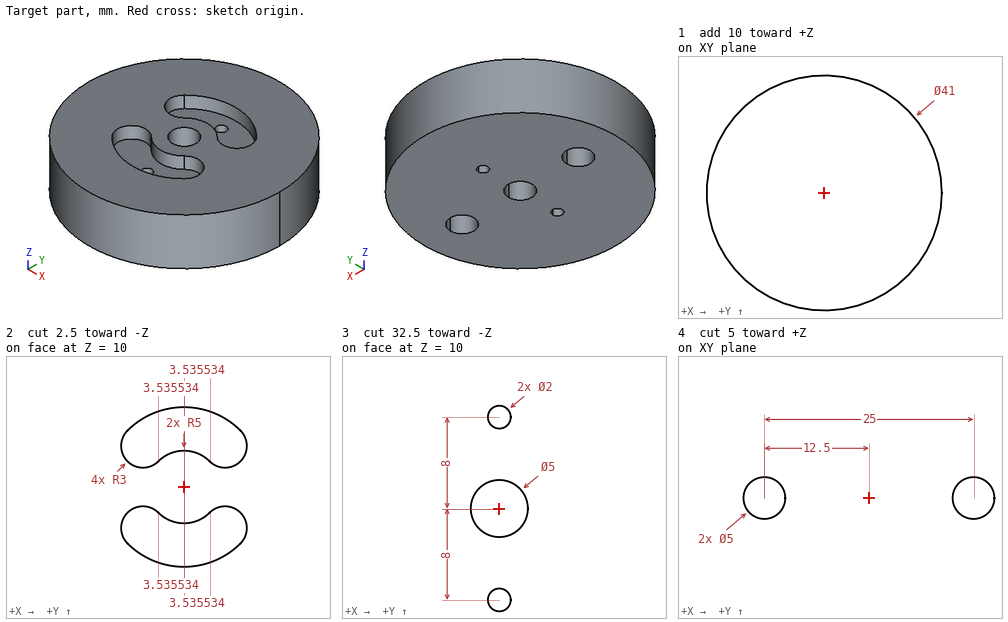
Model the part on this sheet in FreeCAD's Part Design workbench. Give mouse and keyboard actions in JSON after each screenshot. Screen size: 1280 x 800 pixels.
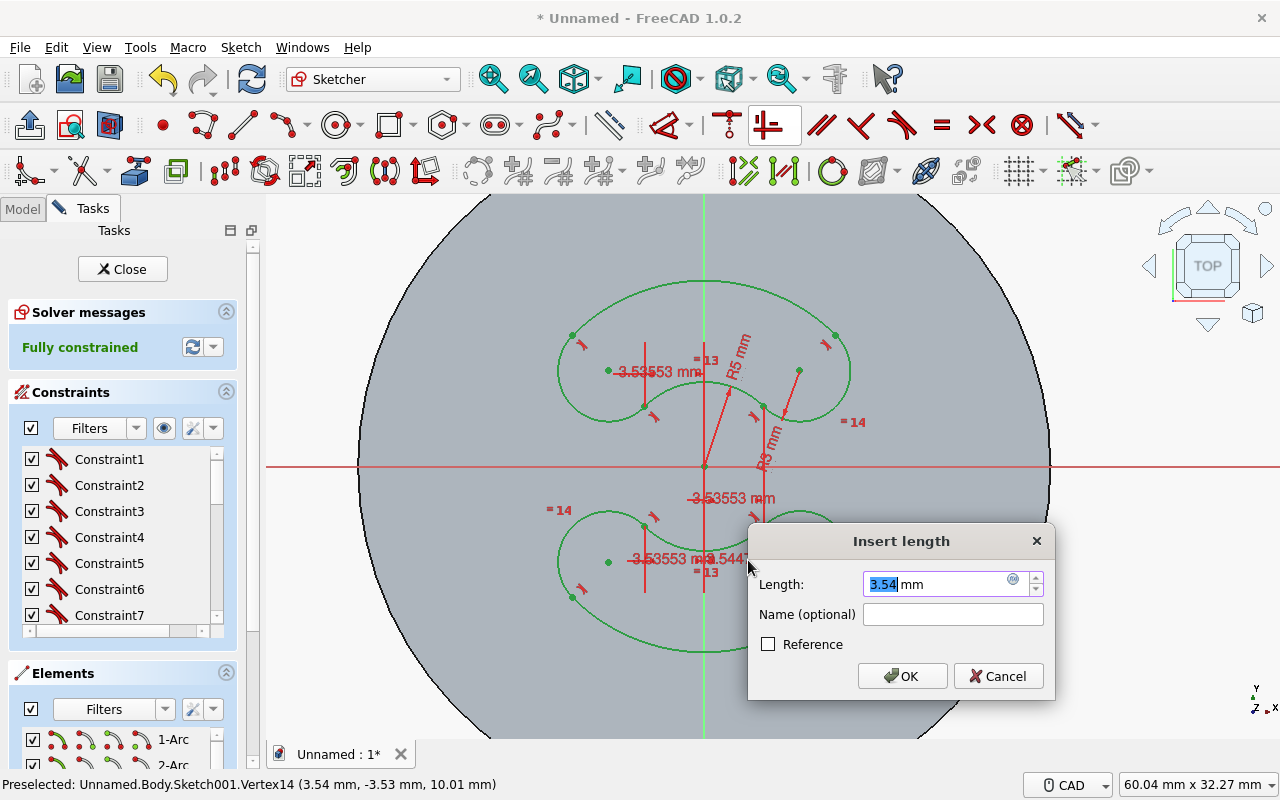
{"action": "type", "text": "3.535534"}
{"action": "key", "text": "Return"}
{"action": "key", "text": "Escape"}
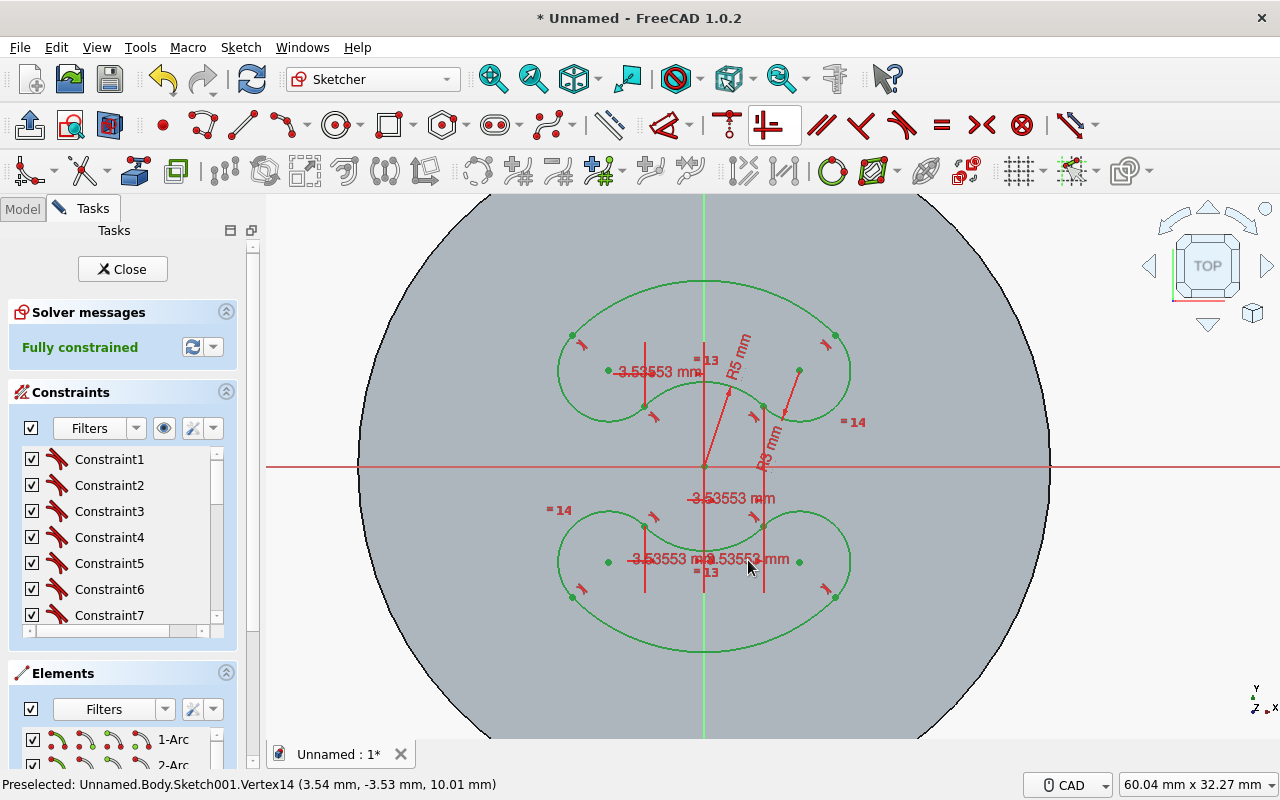
{"action": "left_click", "coordinate": [123, 269]}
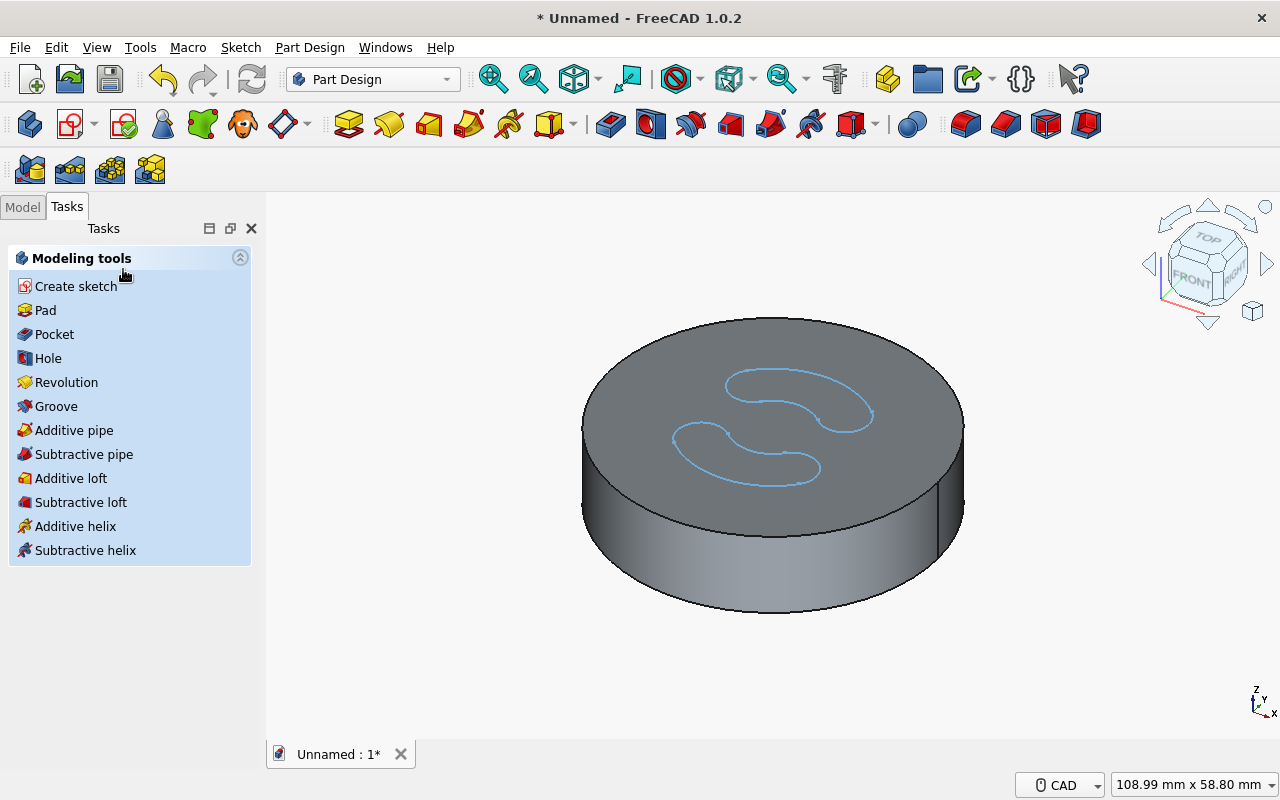
{"action": "left_click", "coordinate": [612, 124]}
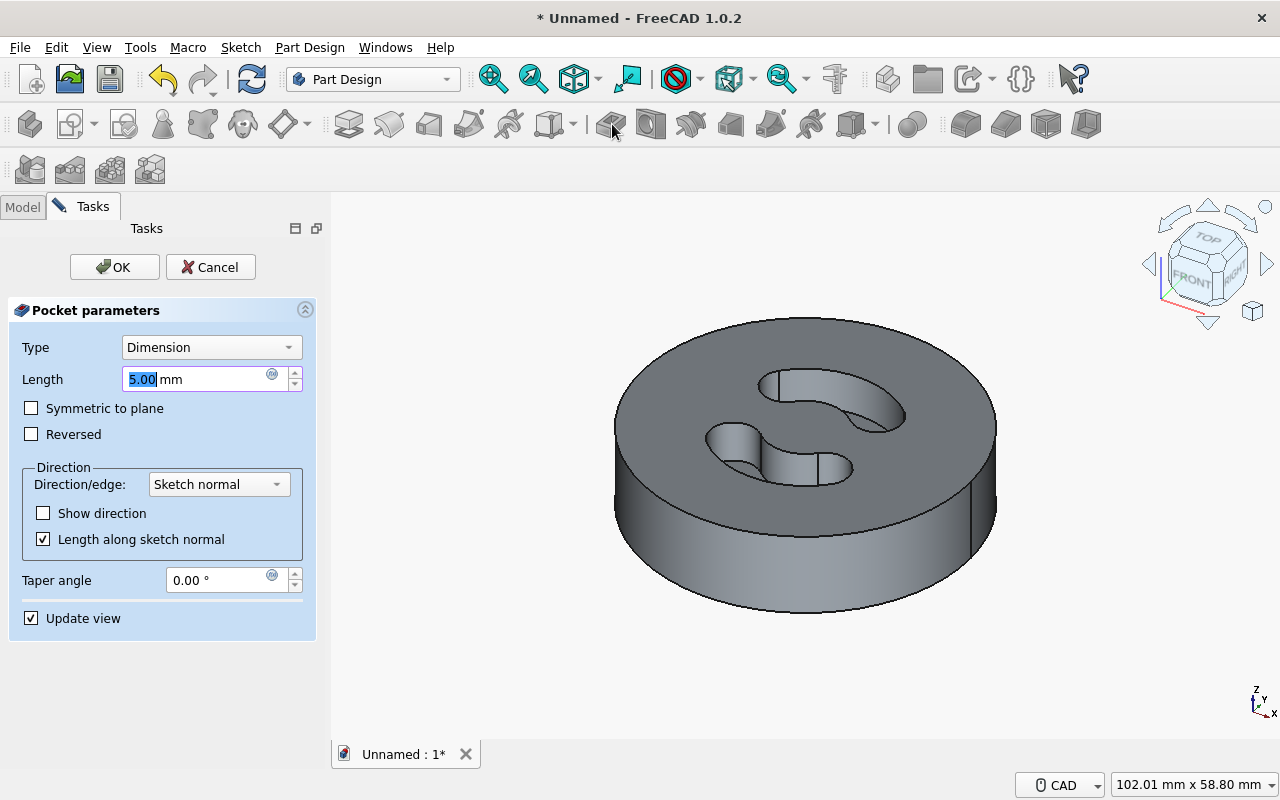
{"action": "type", "text": "2.5"}
{"action": "key", "text": "Tab"}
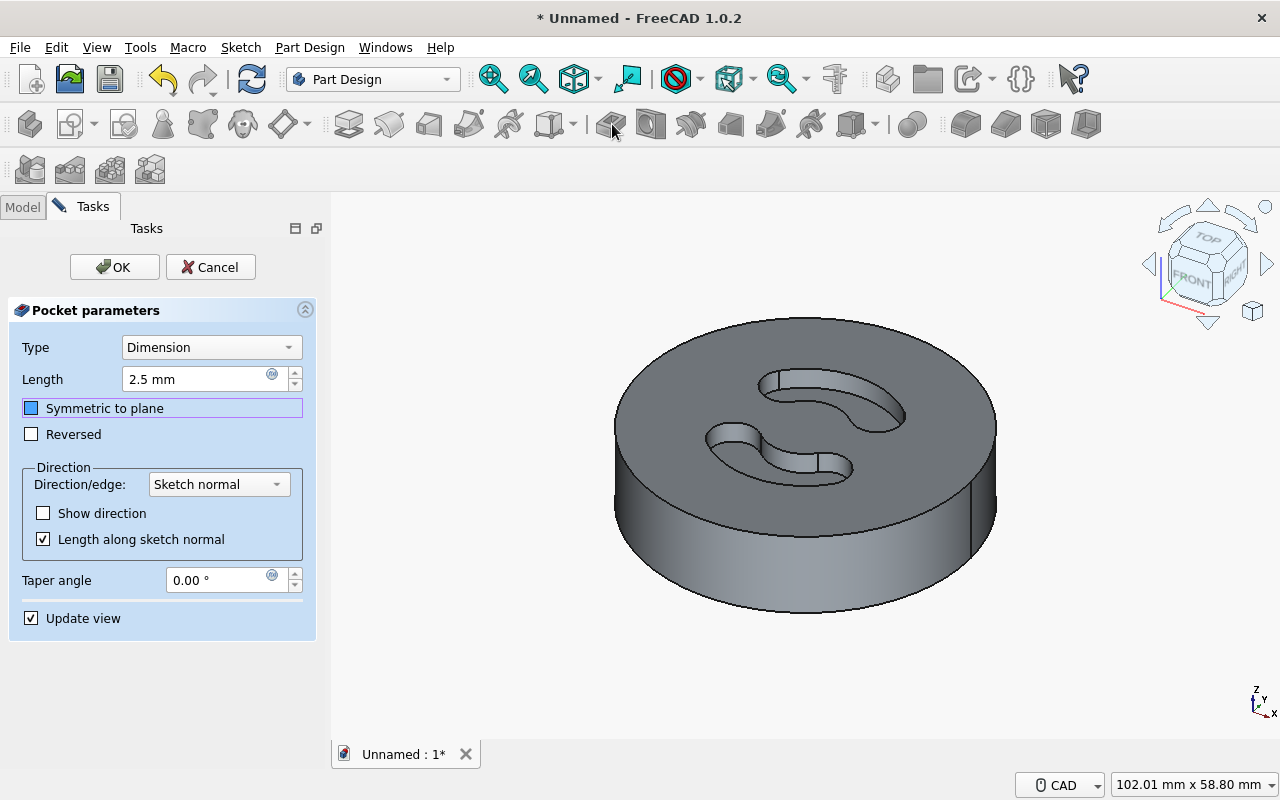
{"action": "left_click", "coordinate": [115, 267]}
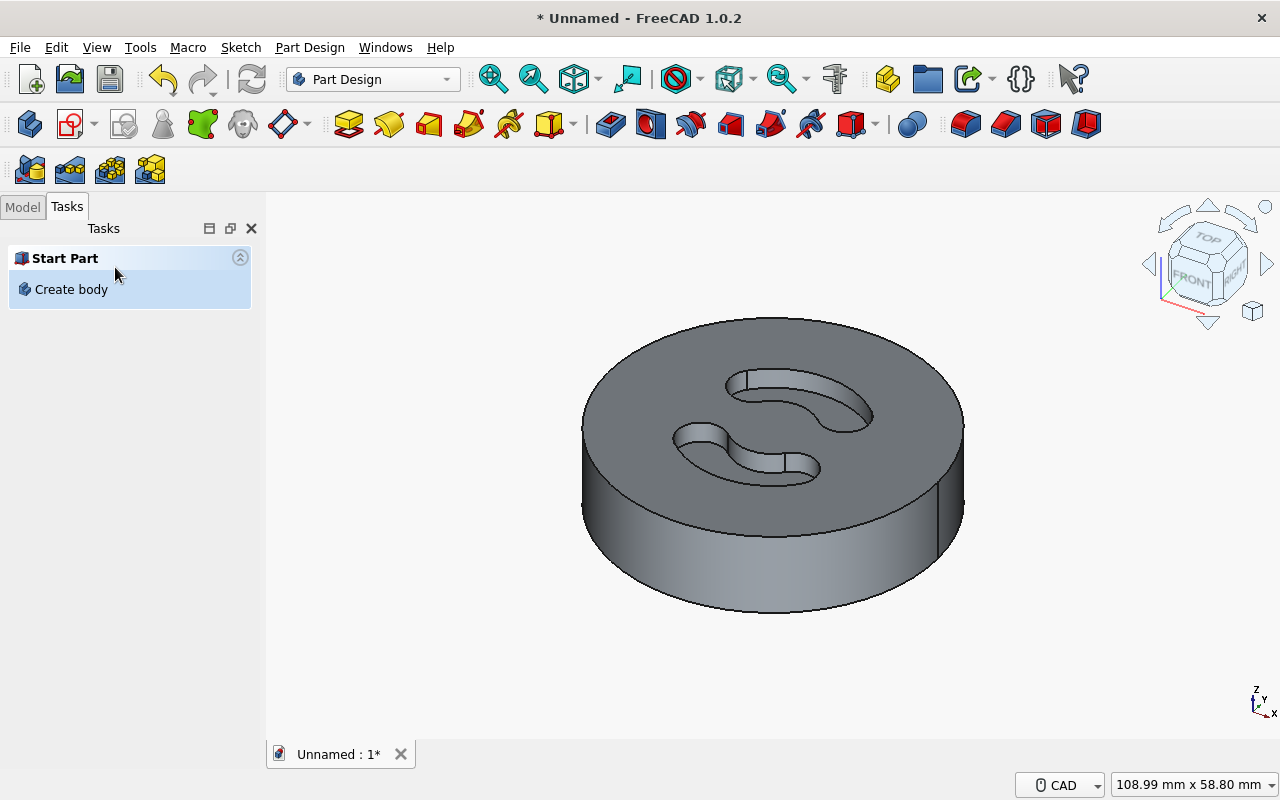
{"action": "left_click", "coordinate": [679, 395]}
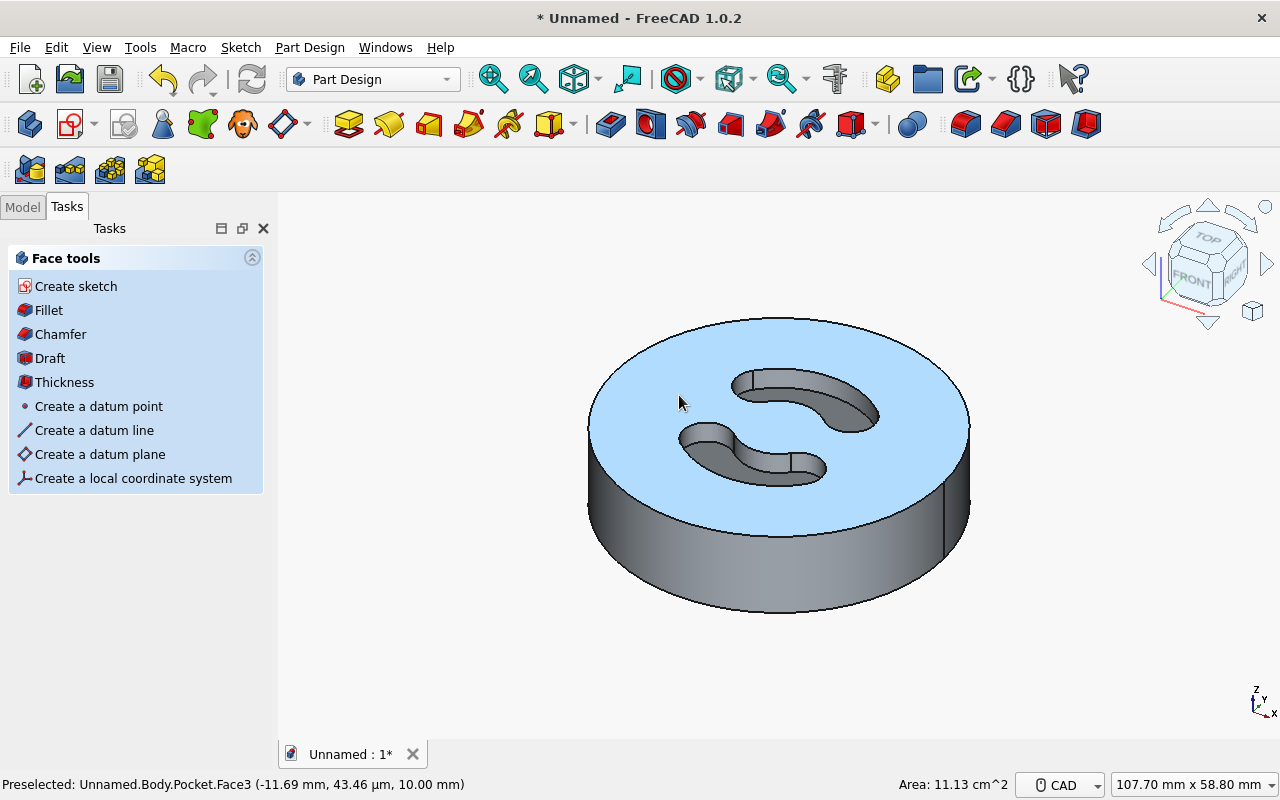
{"action": "left_click", "coordinate": [70, 124]}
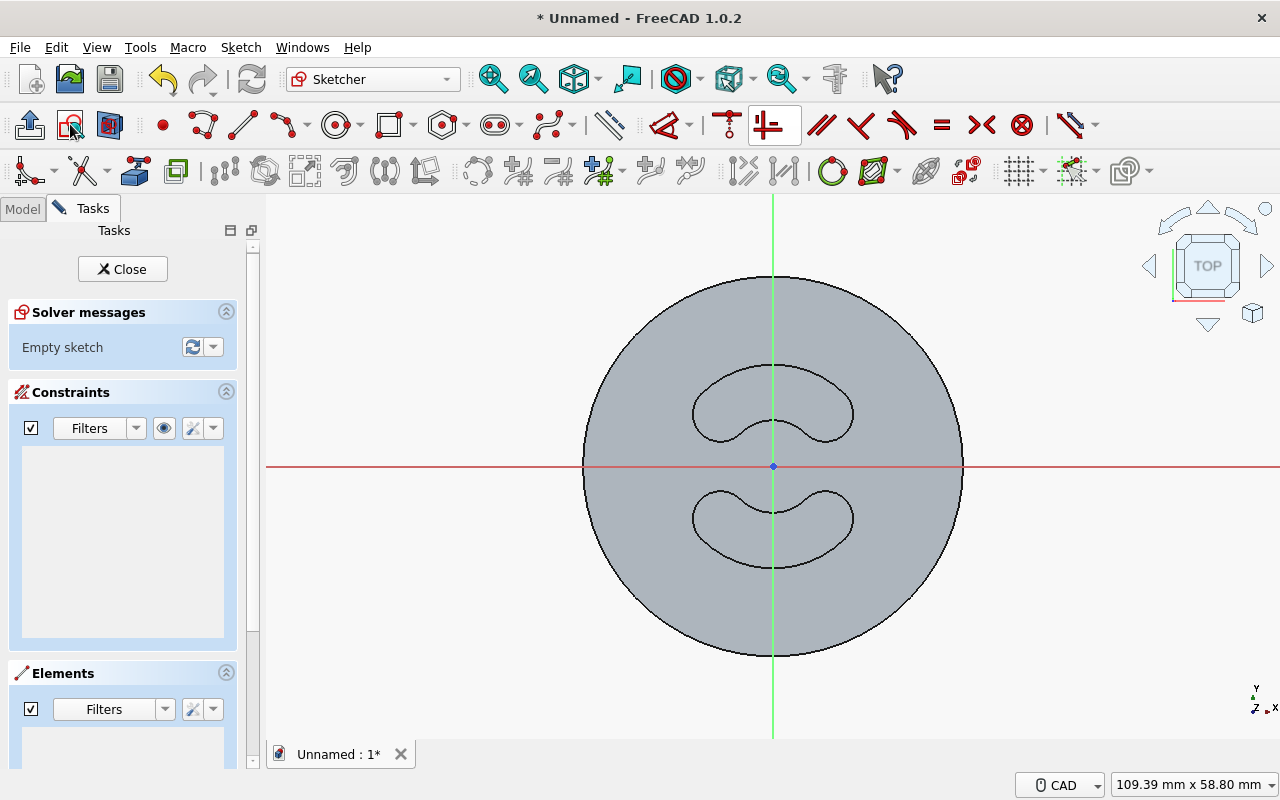
{"action": "scroll", "coordinate": [829, 467], "scroll_direction": "up", "scroll_amount": 4}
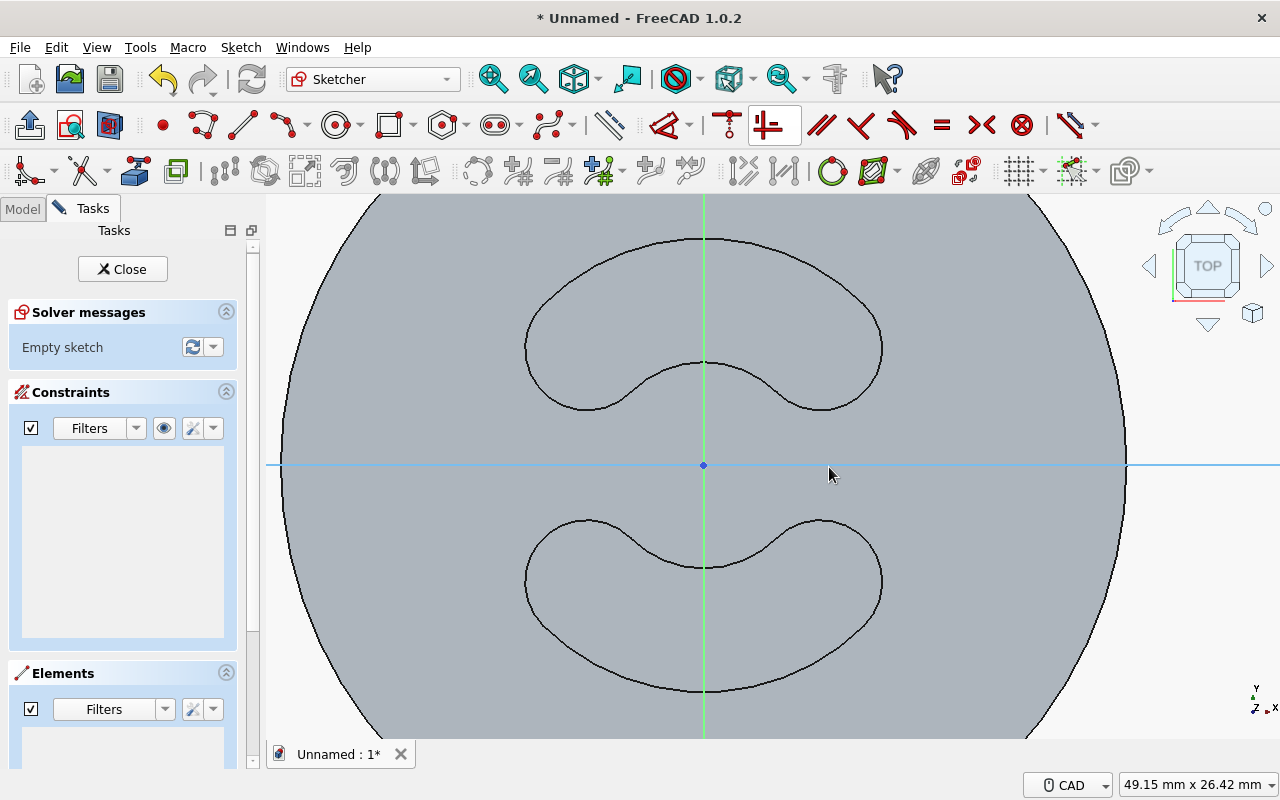
{"action": "key", "text": "g c"}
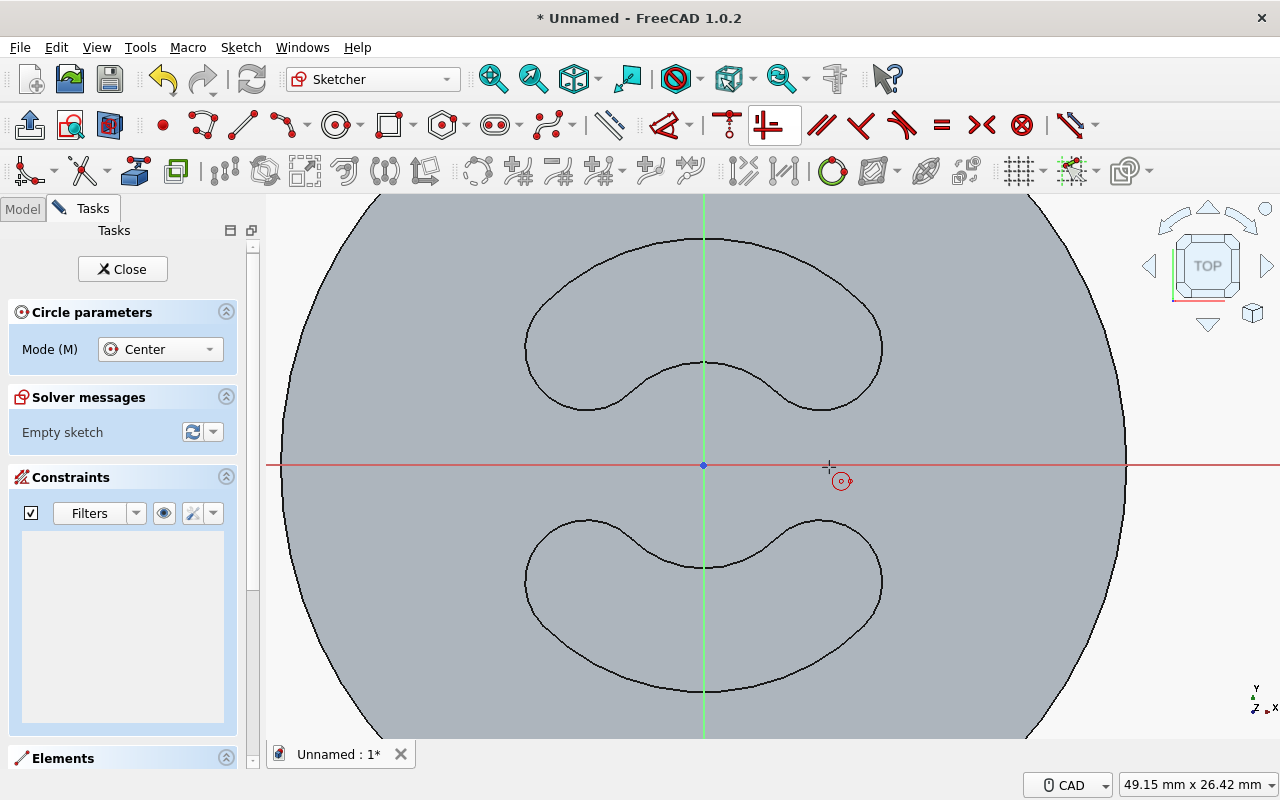
{"action": "left_click", "coordinate": [704, 465]}
{"action": "left_click", "coordinate": [740, 429]}